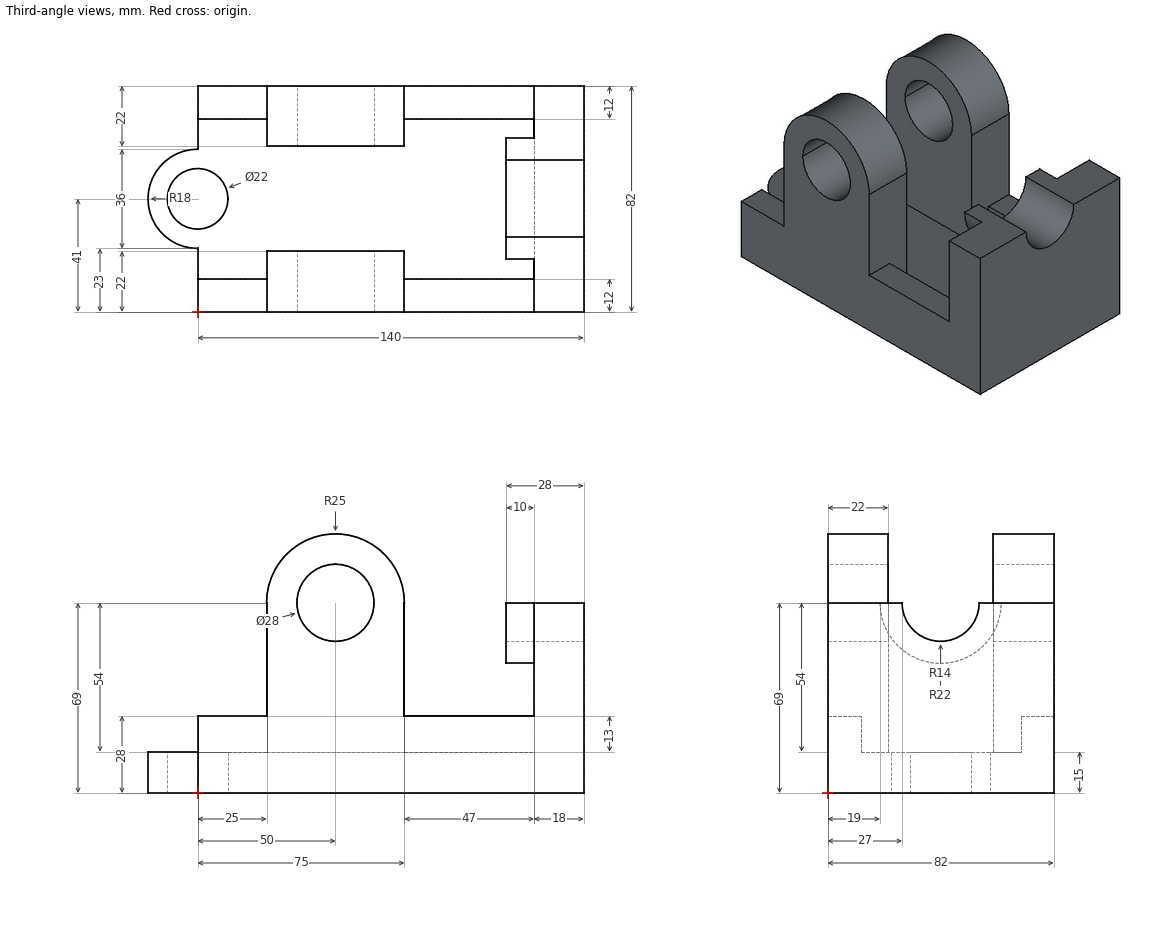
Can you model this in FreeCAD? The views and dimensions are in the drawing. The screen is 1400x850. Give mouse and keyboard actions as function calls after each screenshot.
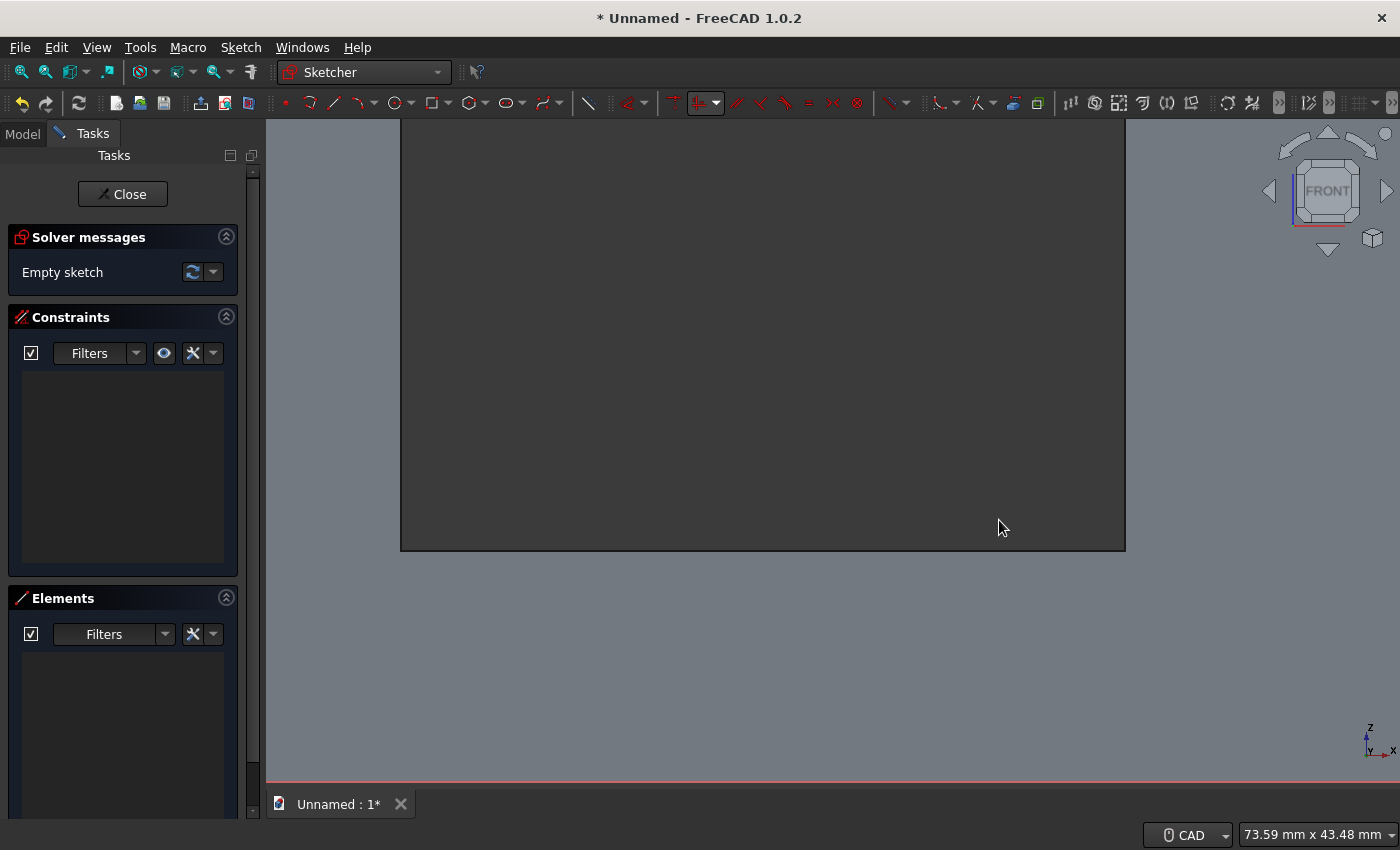
click(432, 104)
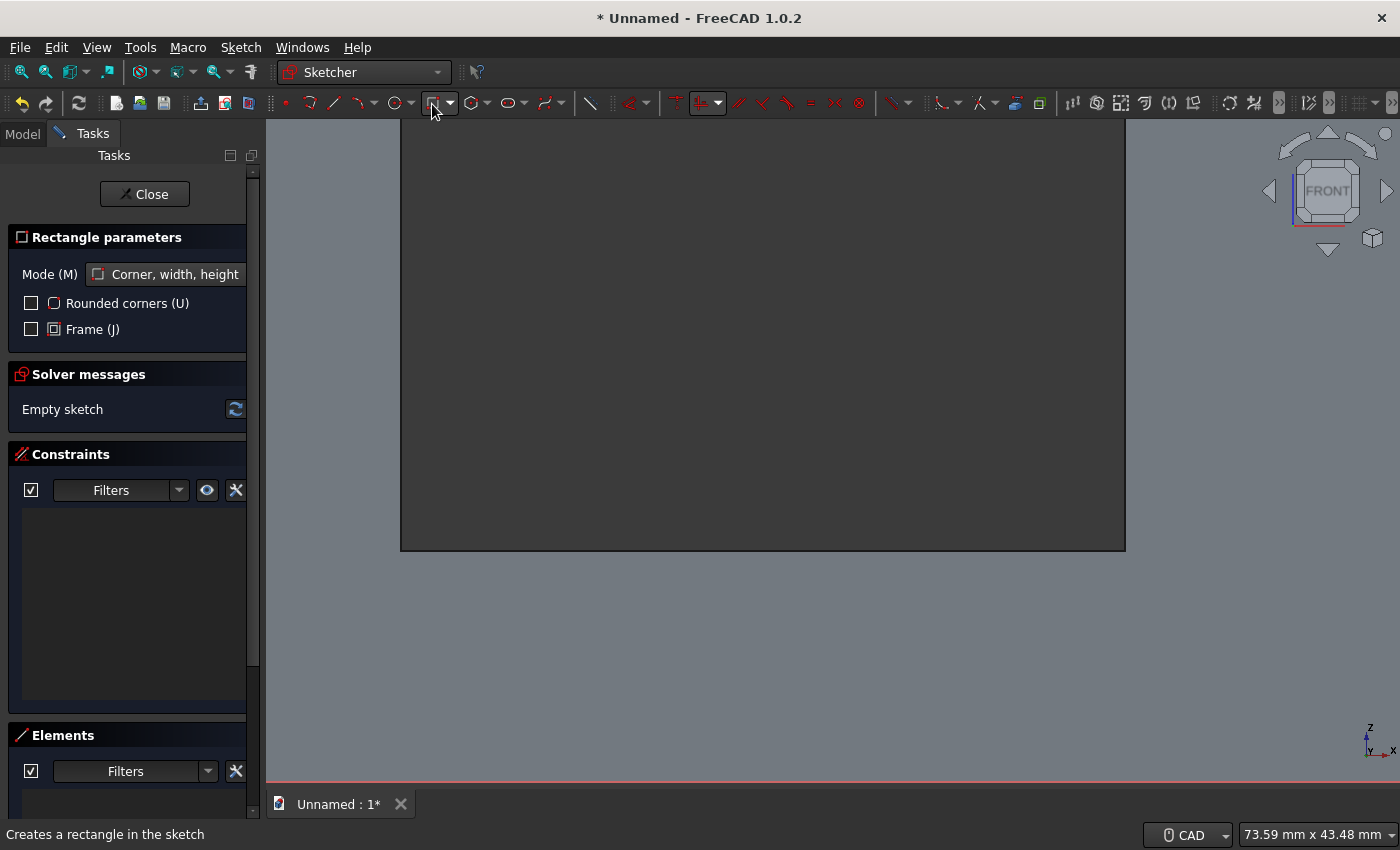
click(401, 351)
click(1125, 551)
key(Escape)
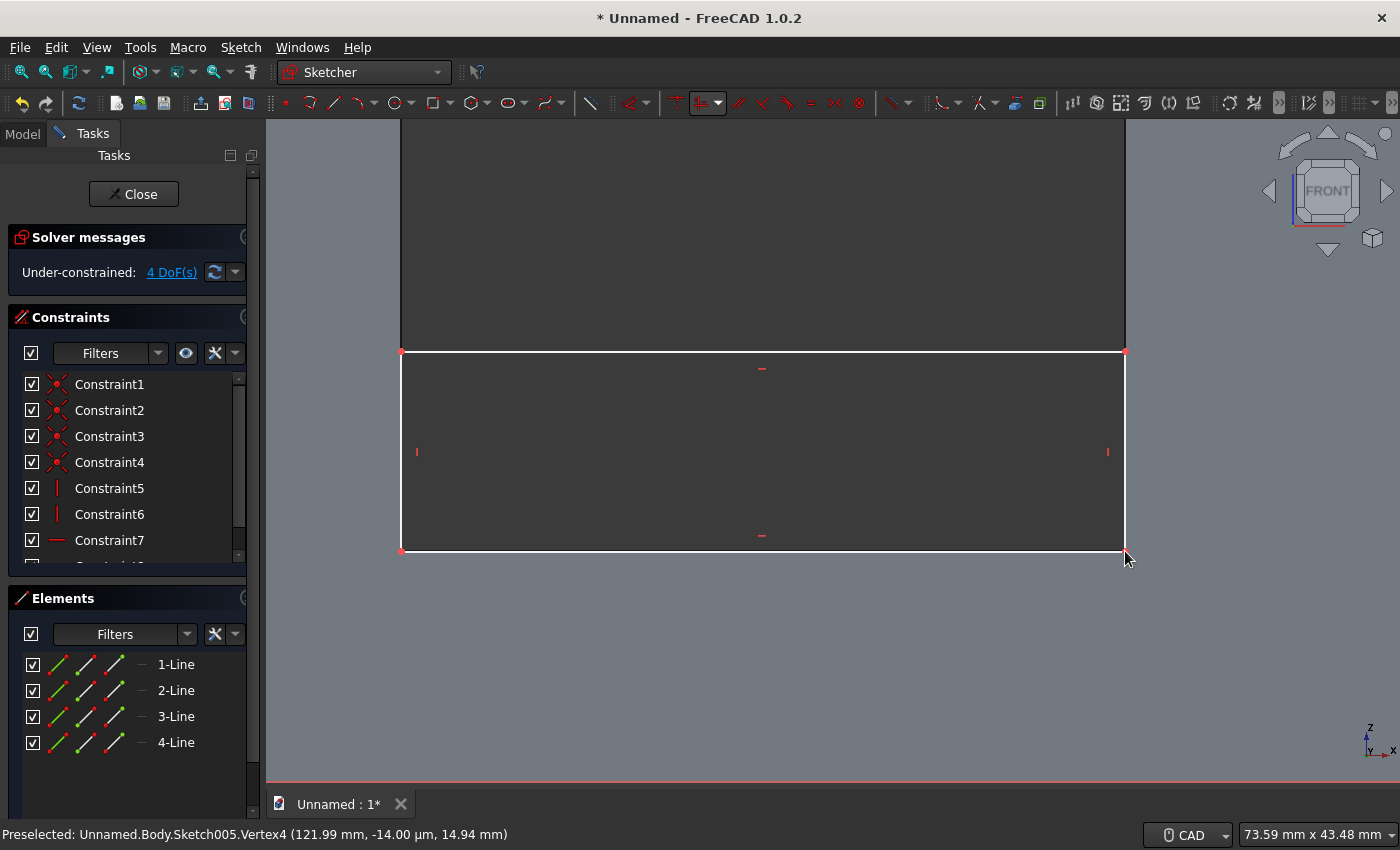
click(630, 104)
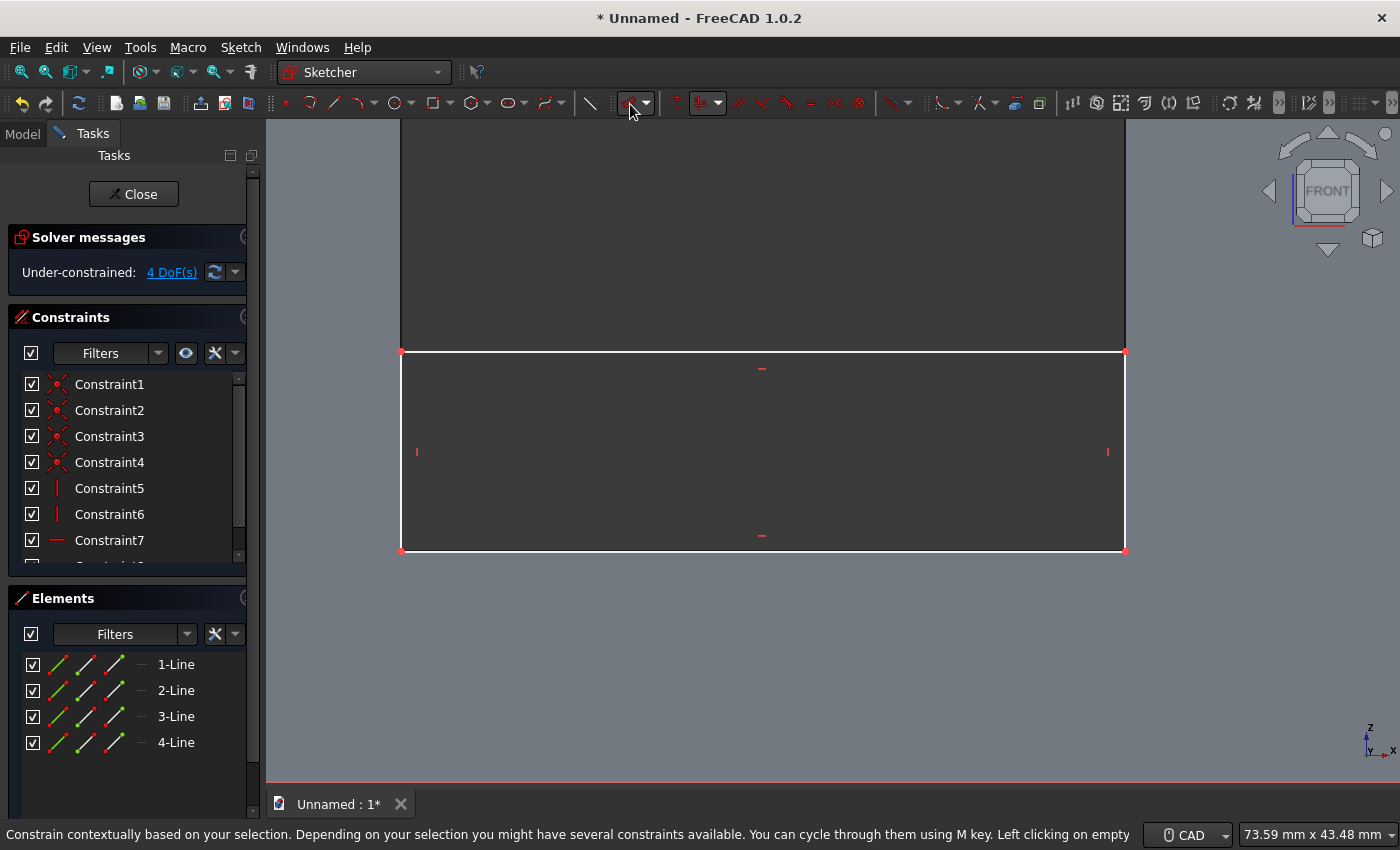
click(401, 412)
click(367, 452)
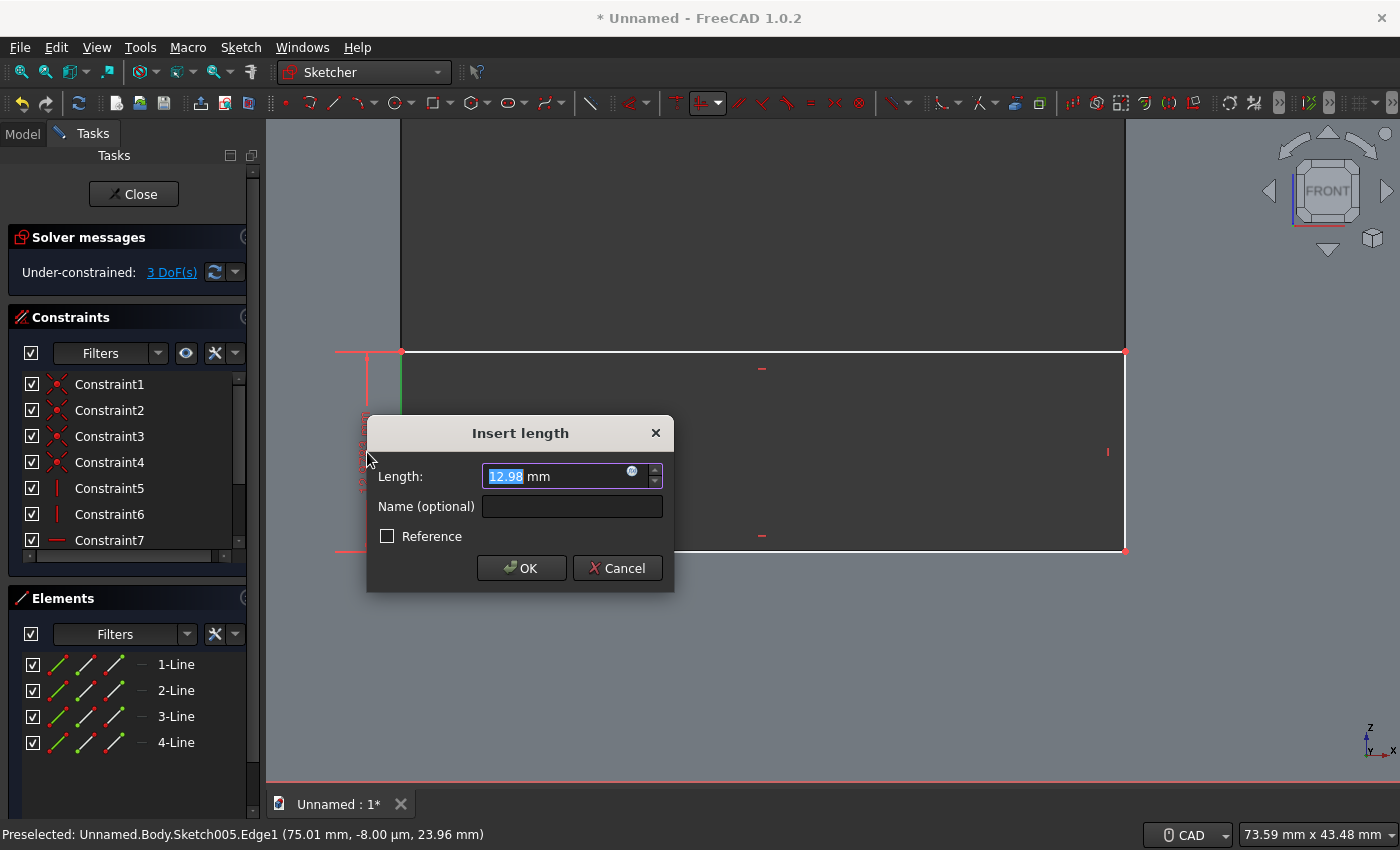
text(13)
key(Return)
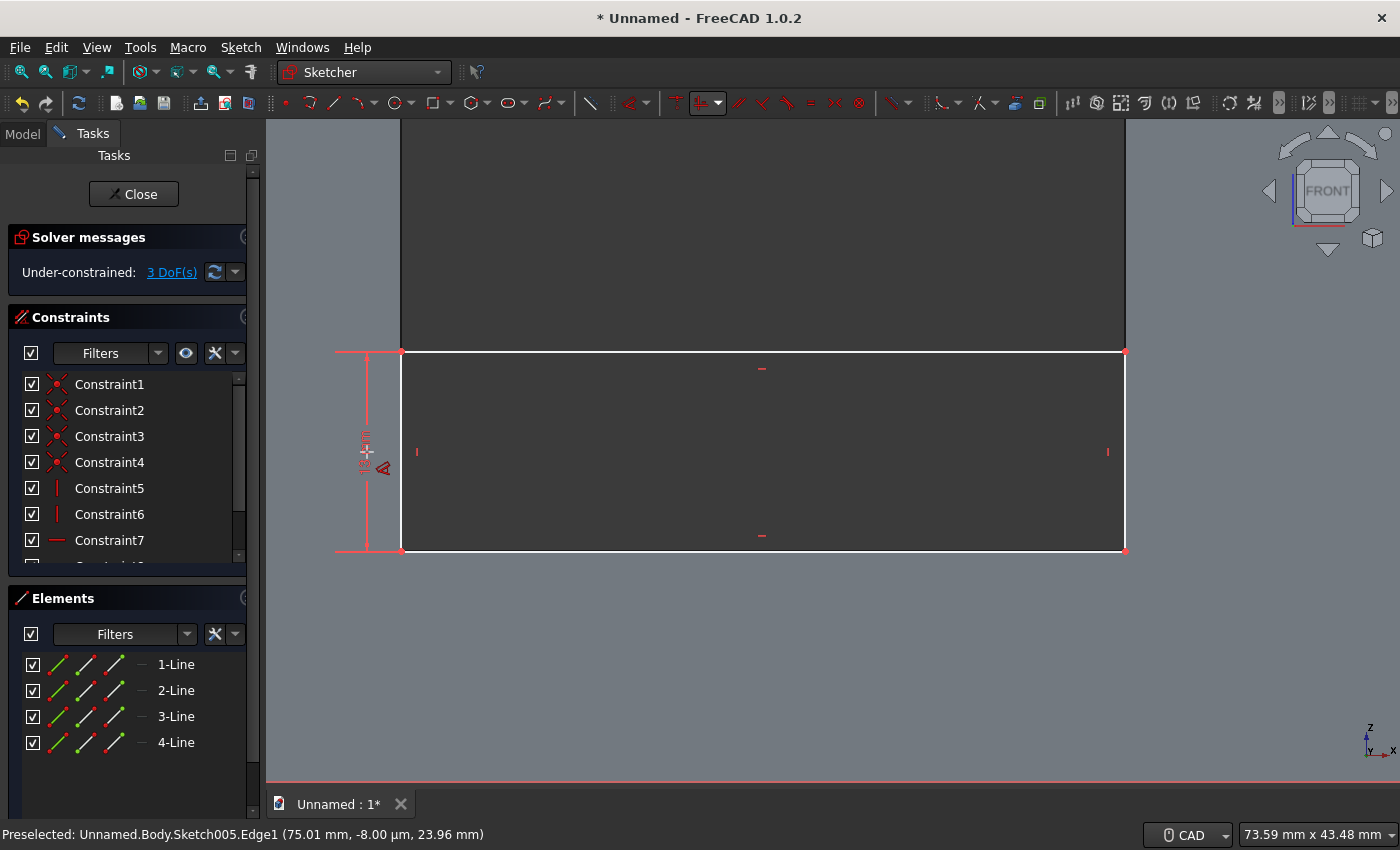
click(618, 552)
click(763, 586)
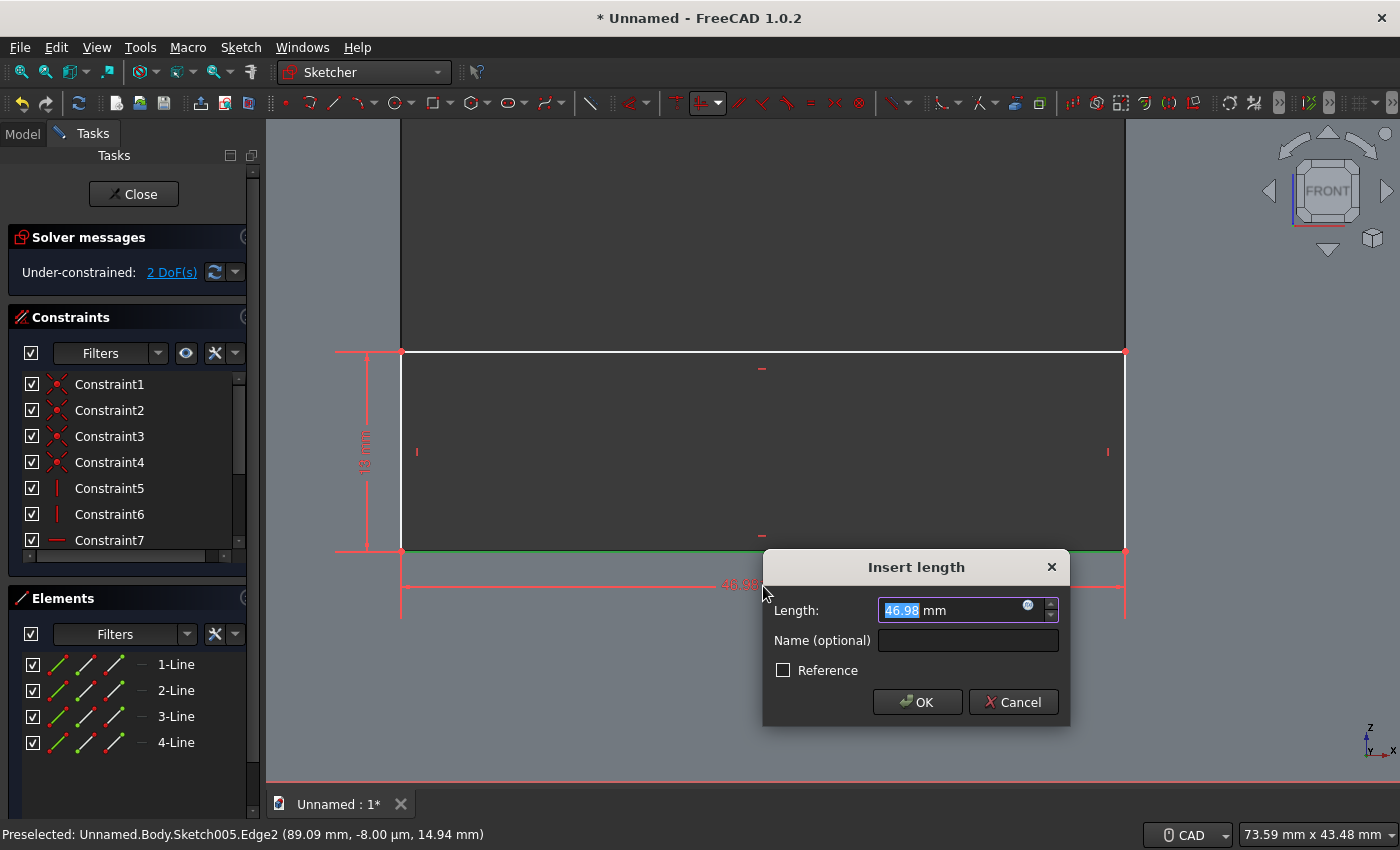
text(47)
key(Return)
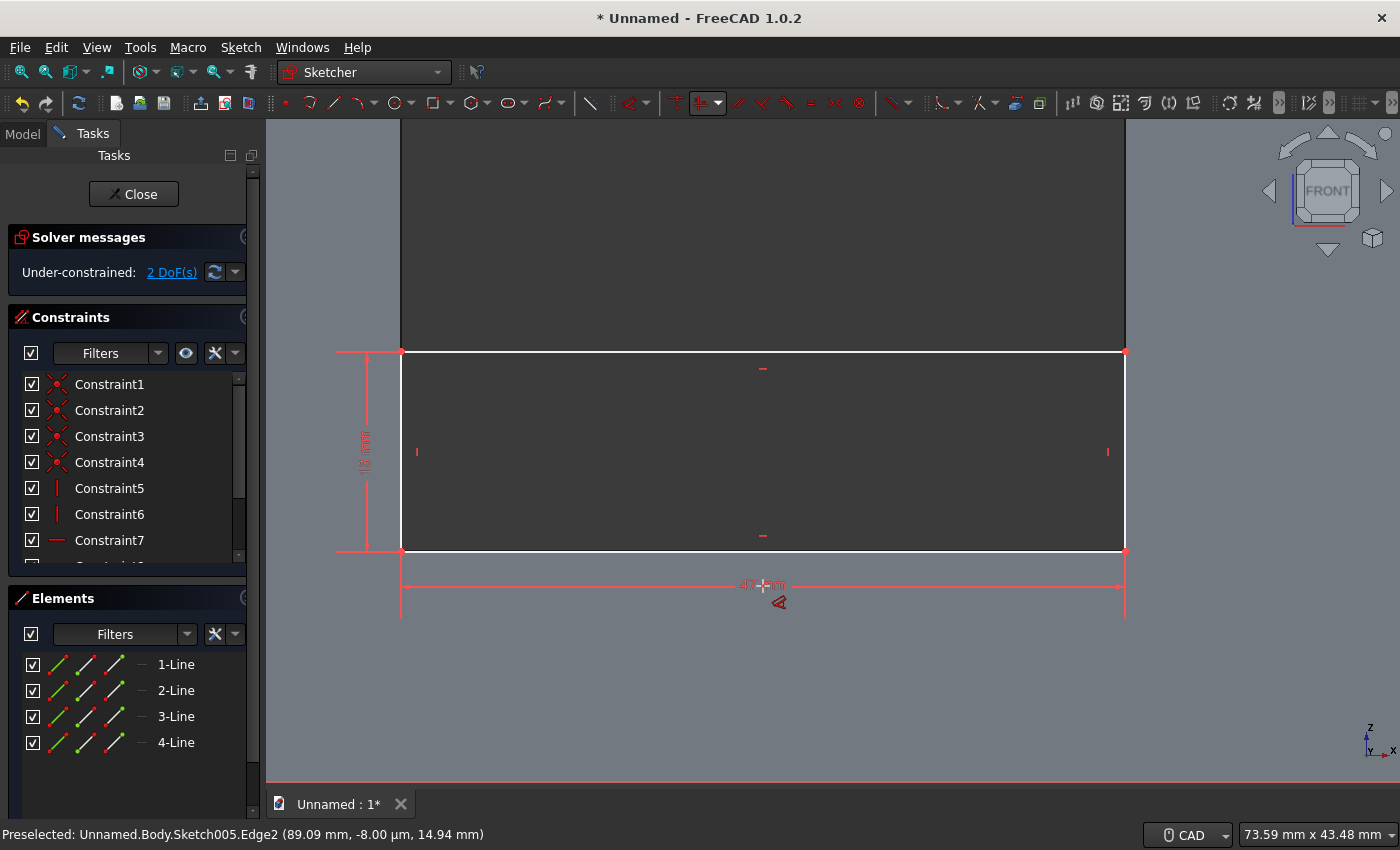
click(401, 352)
click(348, 318)